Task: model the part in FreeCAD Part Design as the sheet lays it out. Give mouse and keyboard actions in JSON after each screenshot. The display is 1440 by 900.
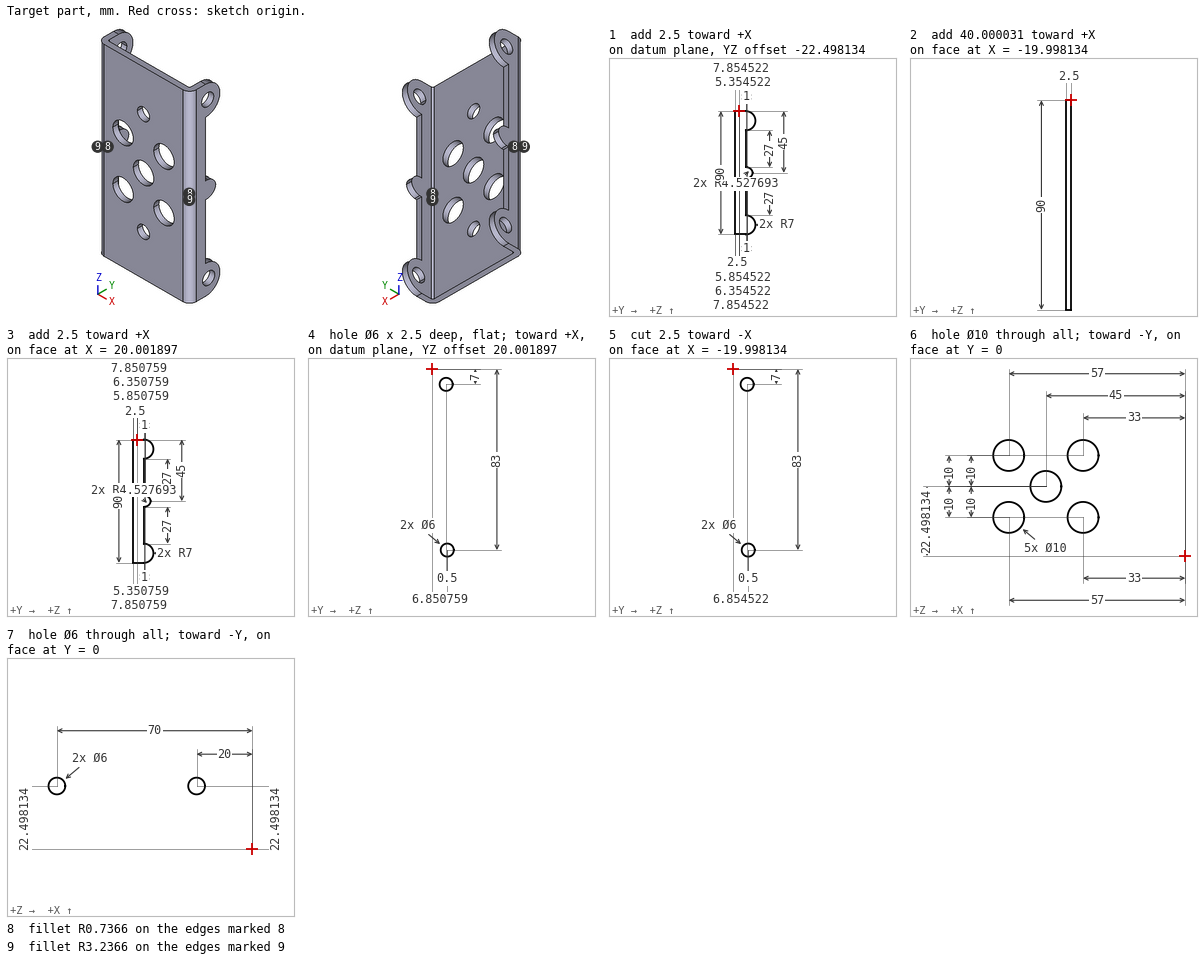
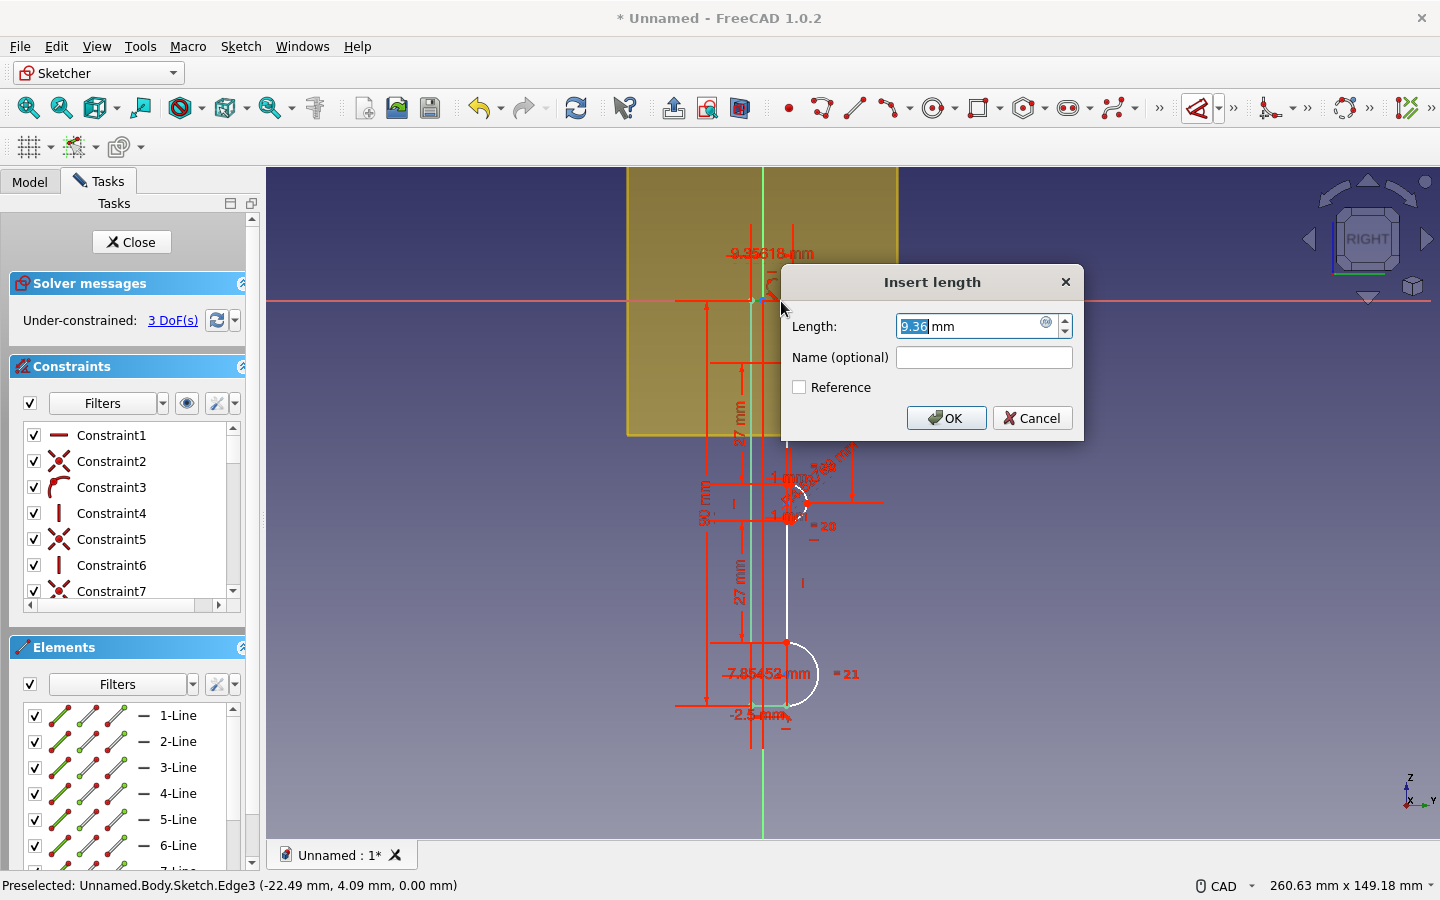
{"action": "type", "text": "7.854522"}
{"action": "key", "text": "Return"}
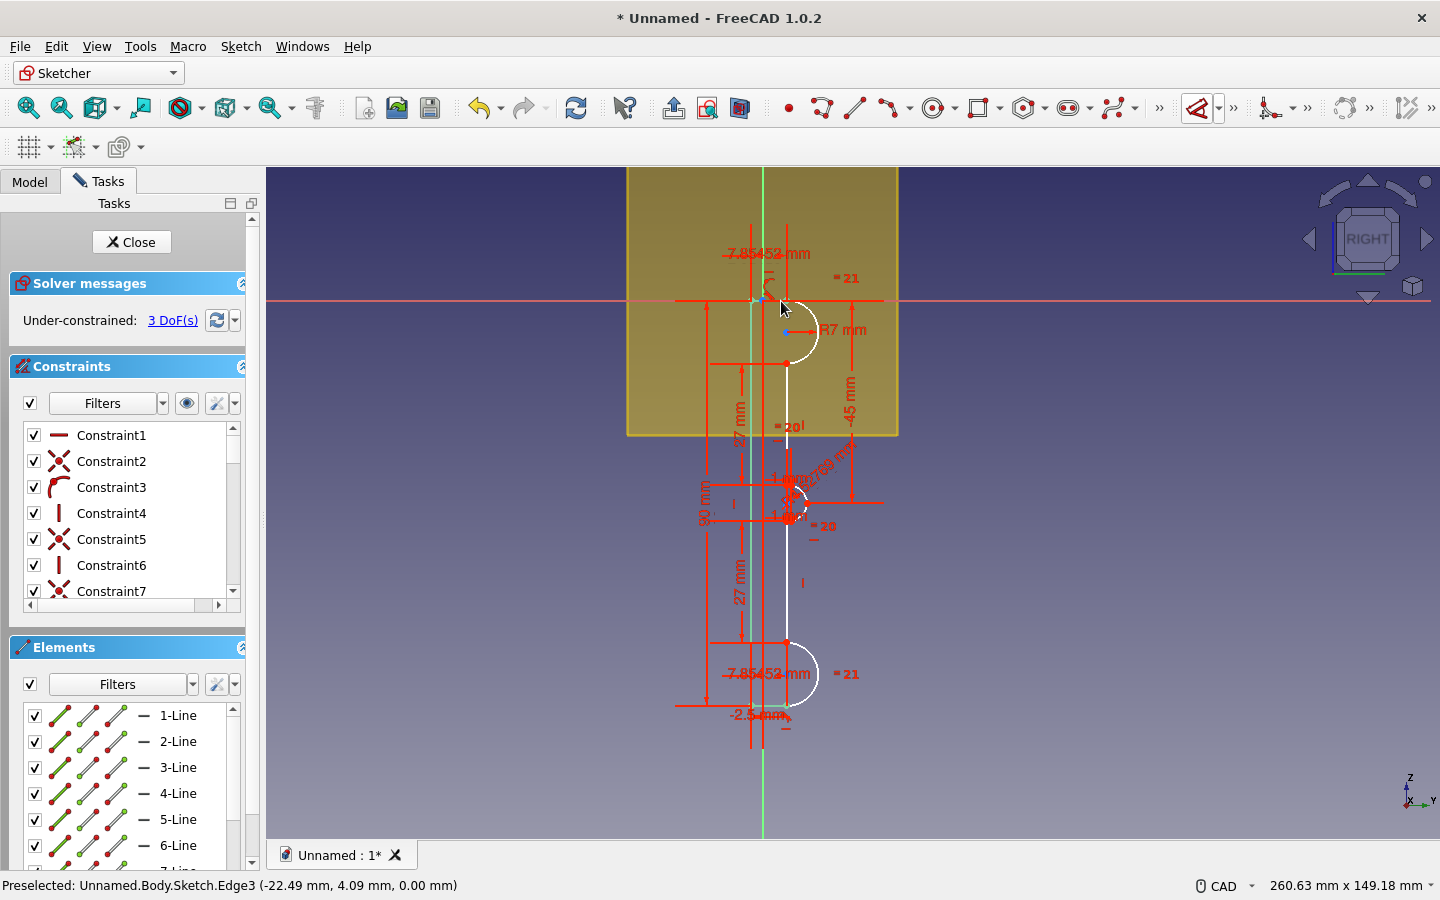
{"action": "scroll", "coordinate": [787, 364], "scroll_direction": "up", "scroll_amount": 3}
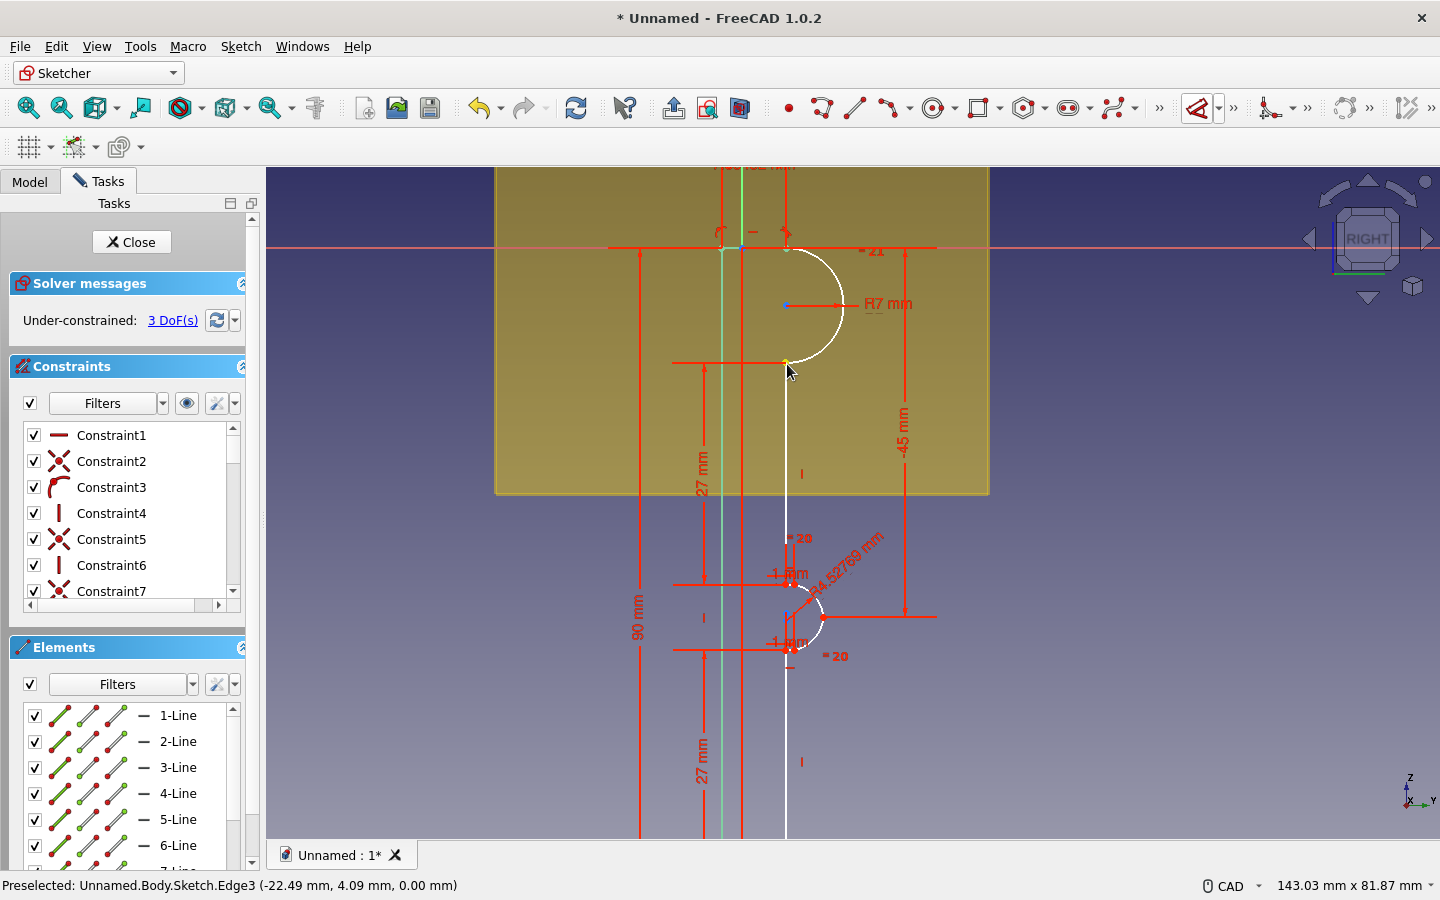
{"action": "left_click", "coordinate": [786, 363]}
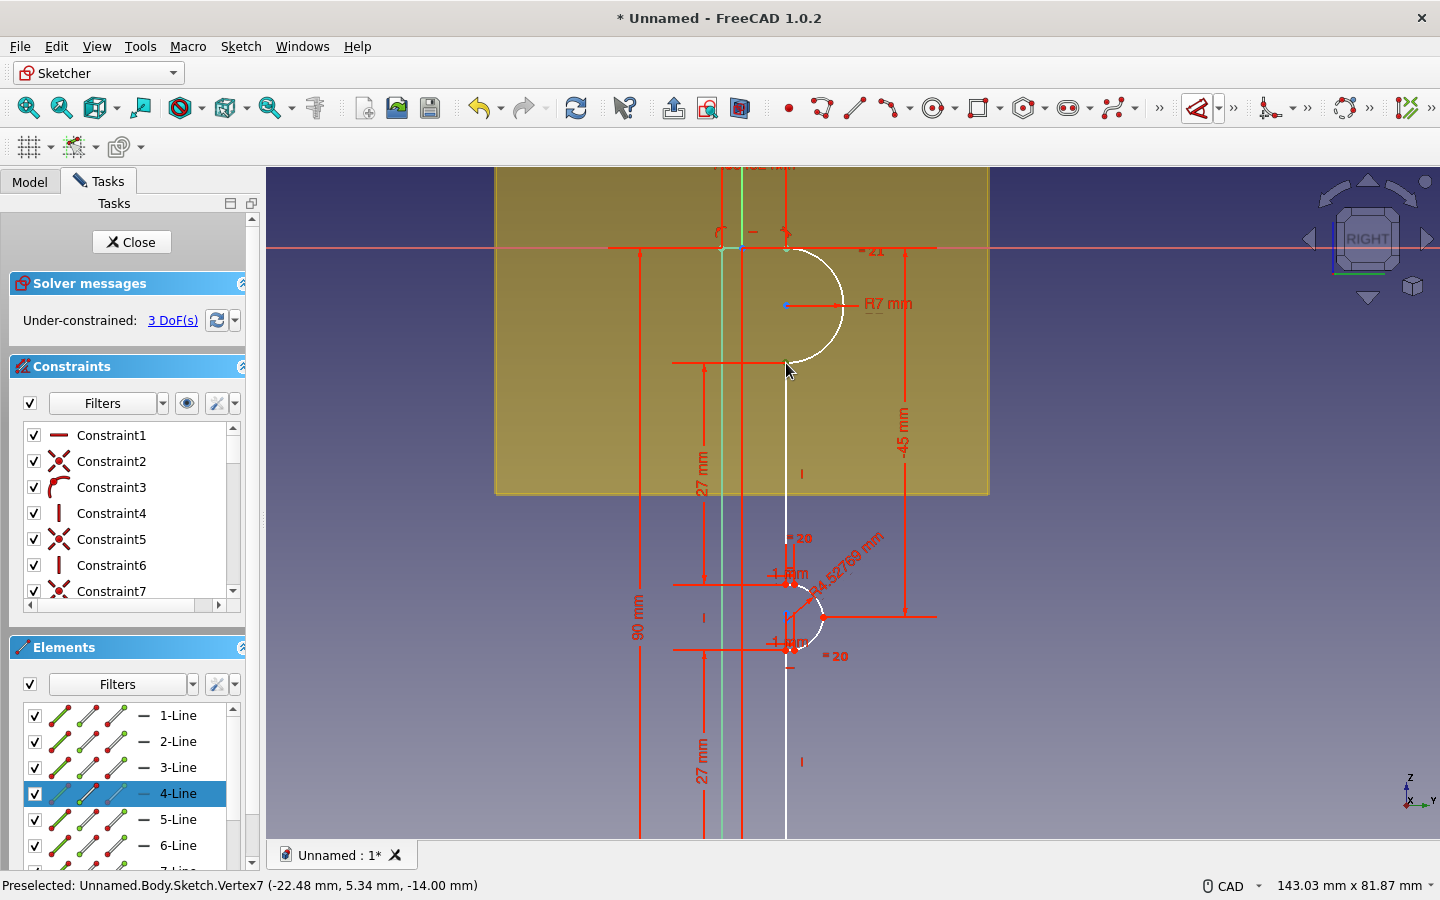
{"action": "left_click", "coordinate": [1218, 108]}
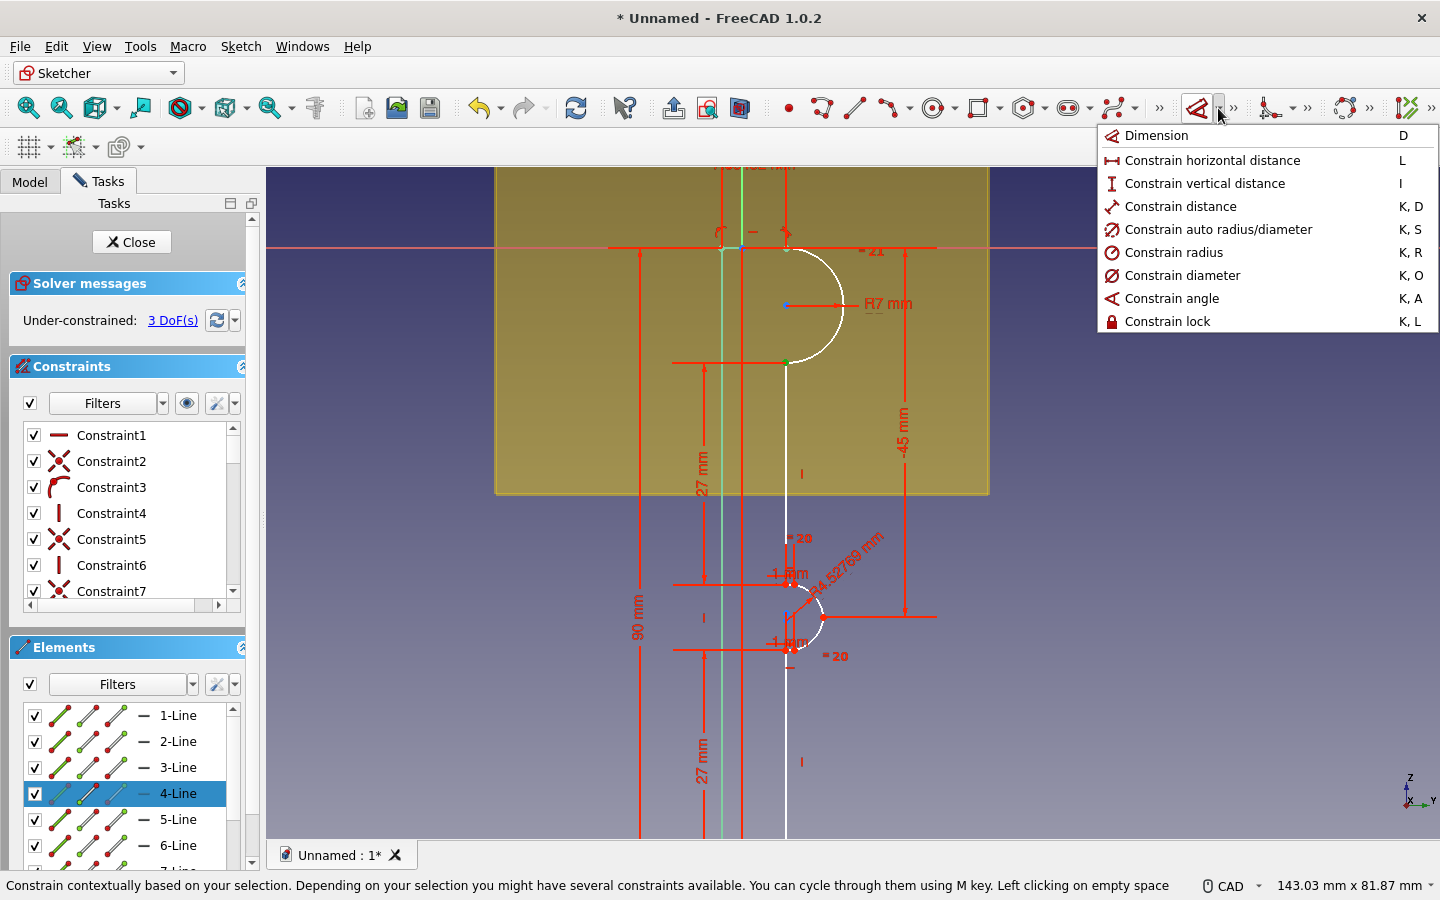
{"action": "left_click", "coordinate": [1268, 160]}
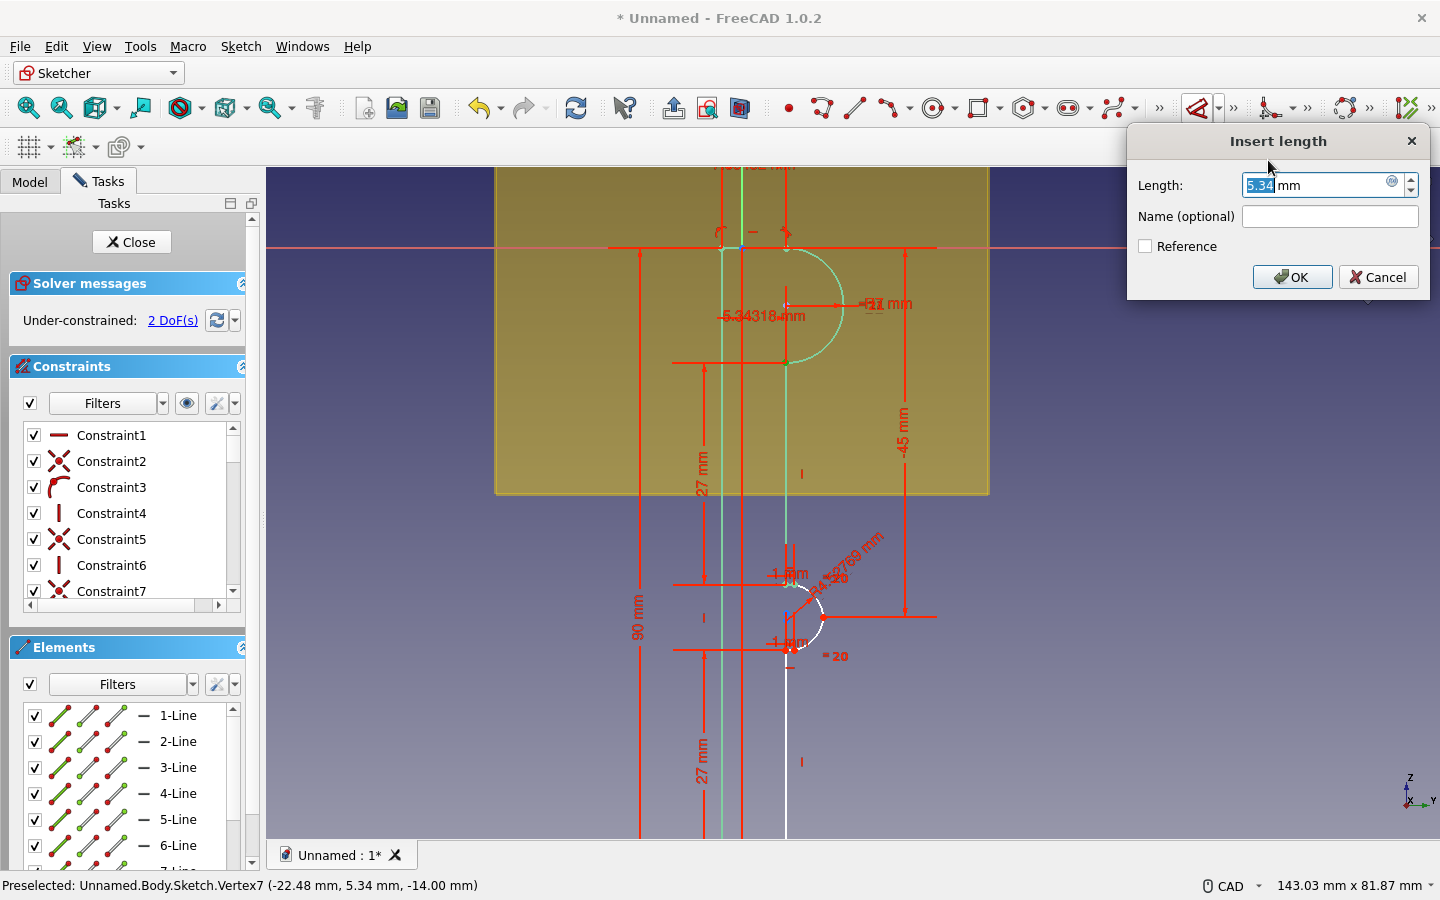
{"action": "type", "text": "5.354522"}
{"action": "key", "text": "Return"}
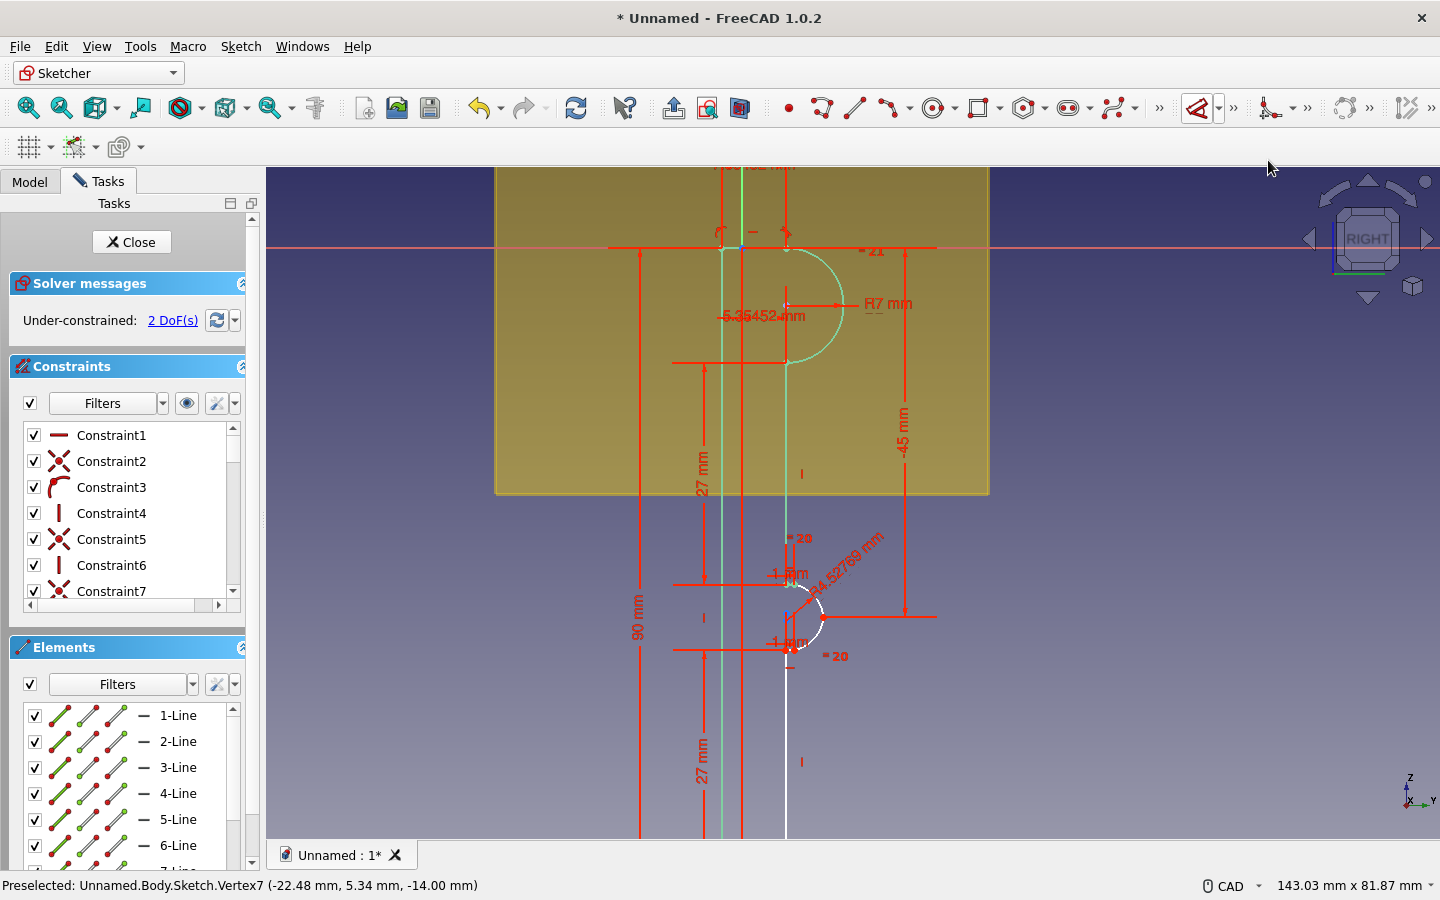
{"action": "scroll", "coordinate": [794, 650], "scroll_direction": "up", "scroll_amount": 2}